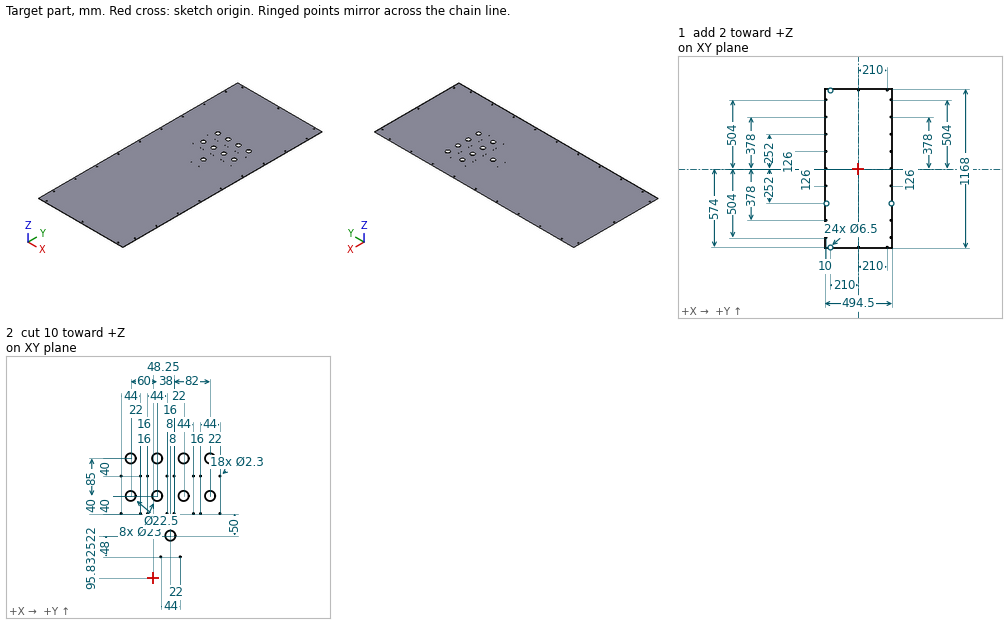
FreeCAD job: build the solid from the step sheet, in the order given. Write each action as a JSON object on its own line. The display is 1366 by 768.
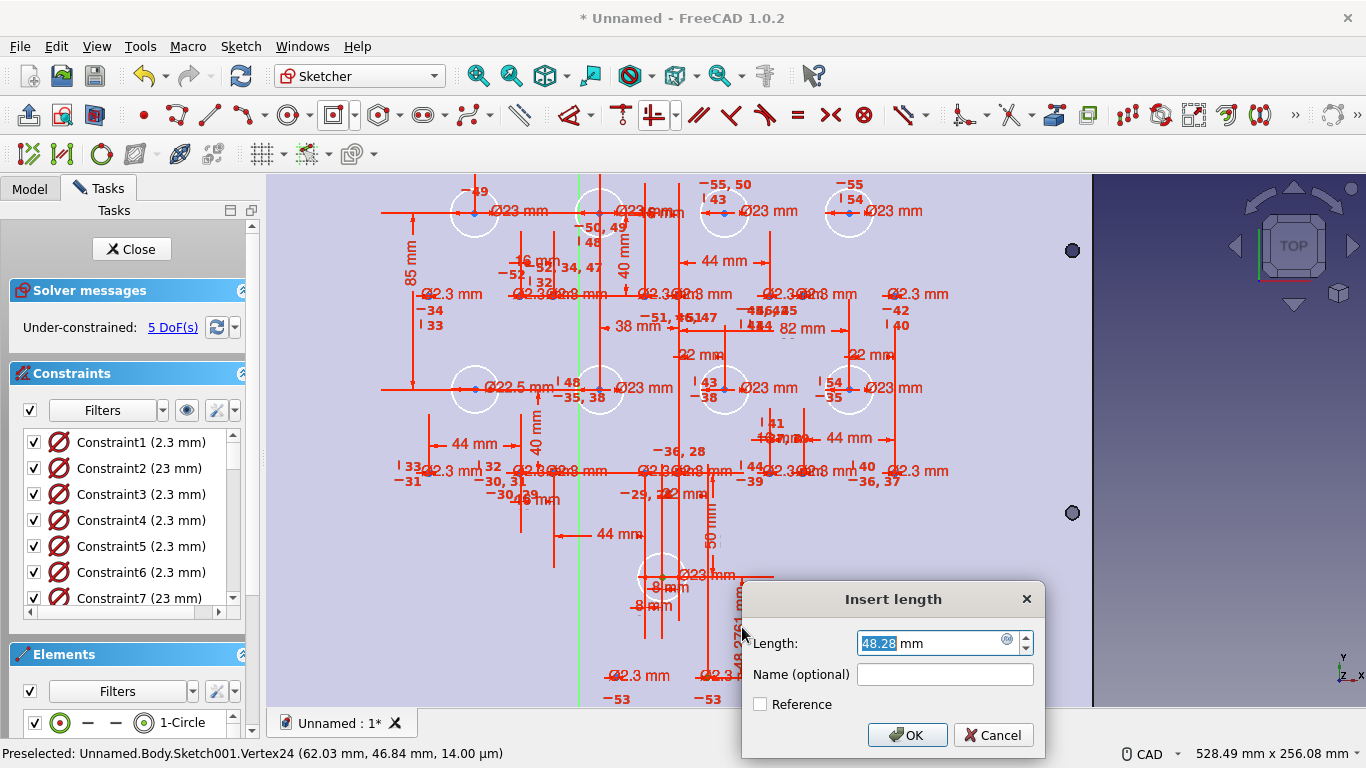
{"action": "type", "text": "48"}
{"action": "key", "text": "Return"}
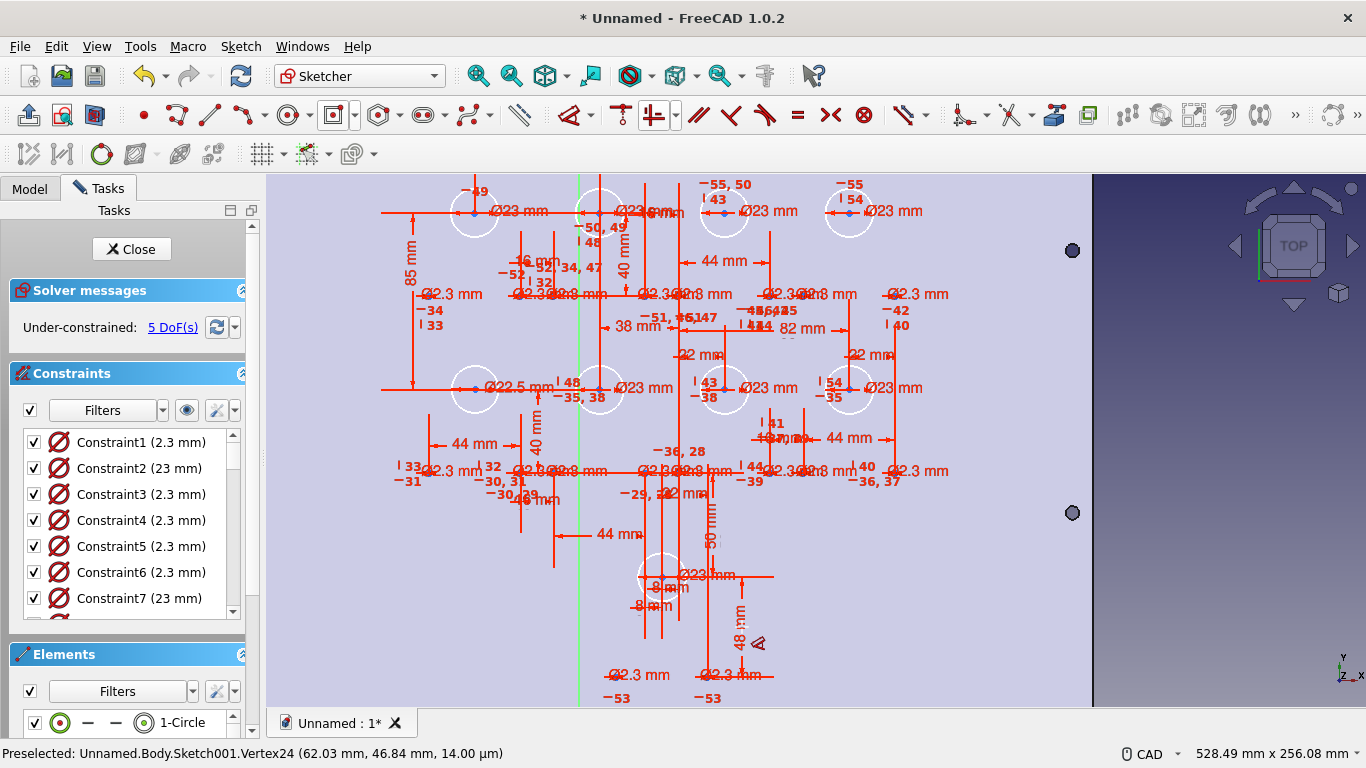
{"action": "left_click", "coordinate": [708, 677]}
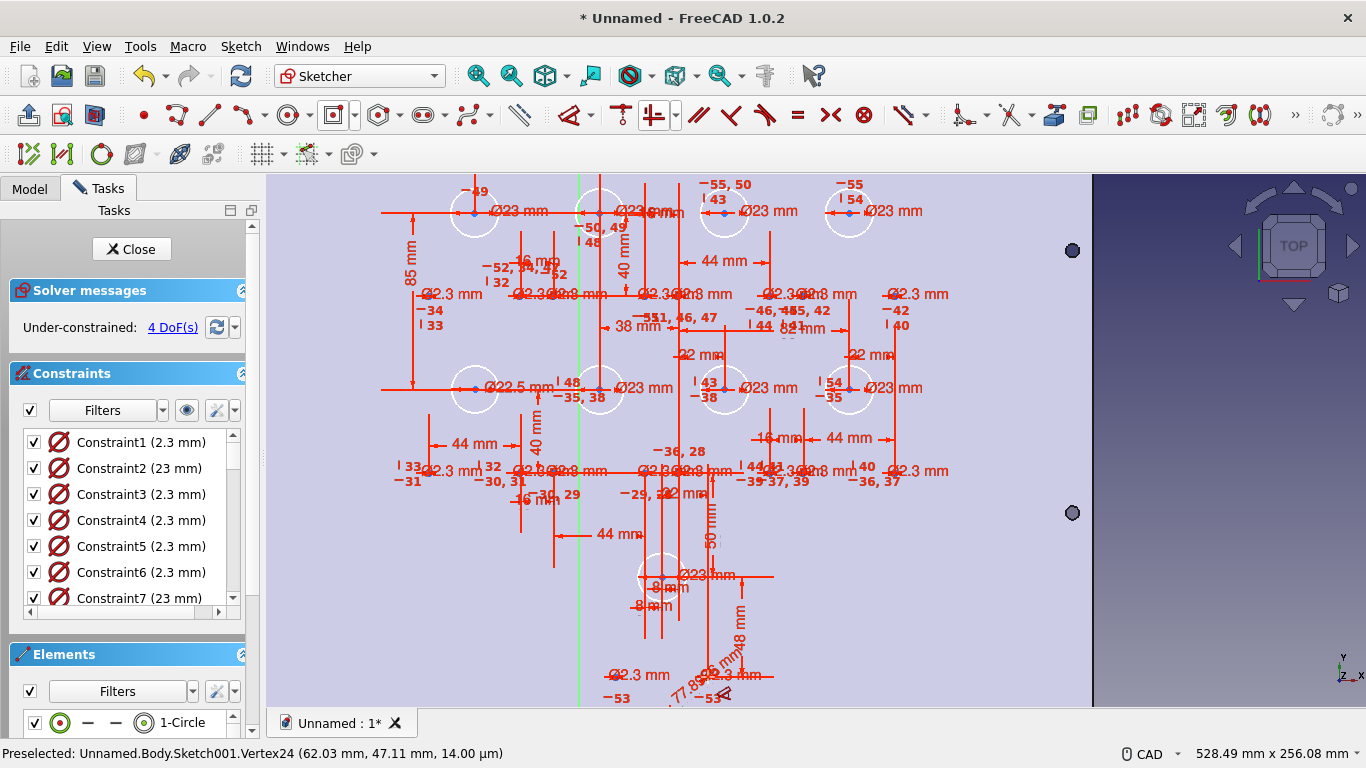
{"action": "left_click", "coordinate": [617, 677]}
{"action": "left_click", "coordinate": [662, 643]}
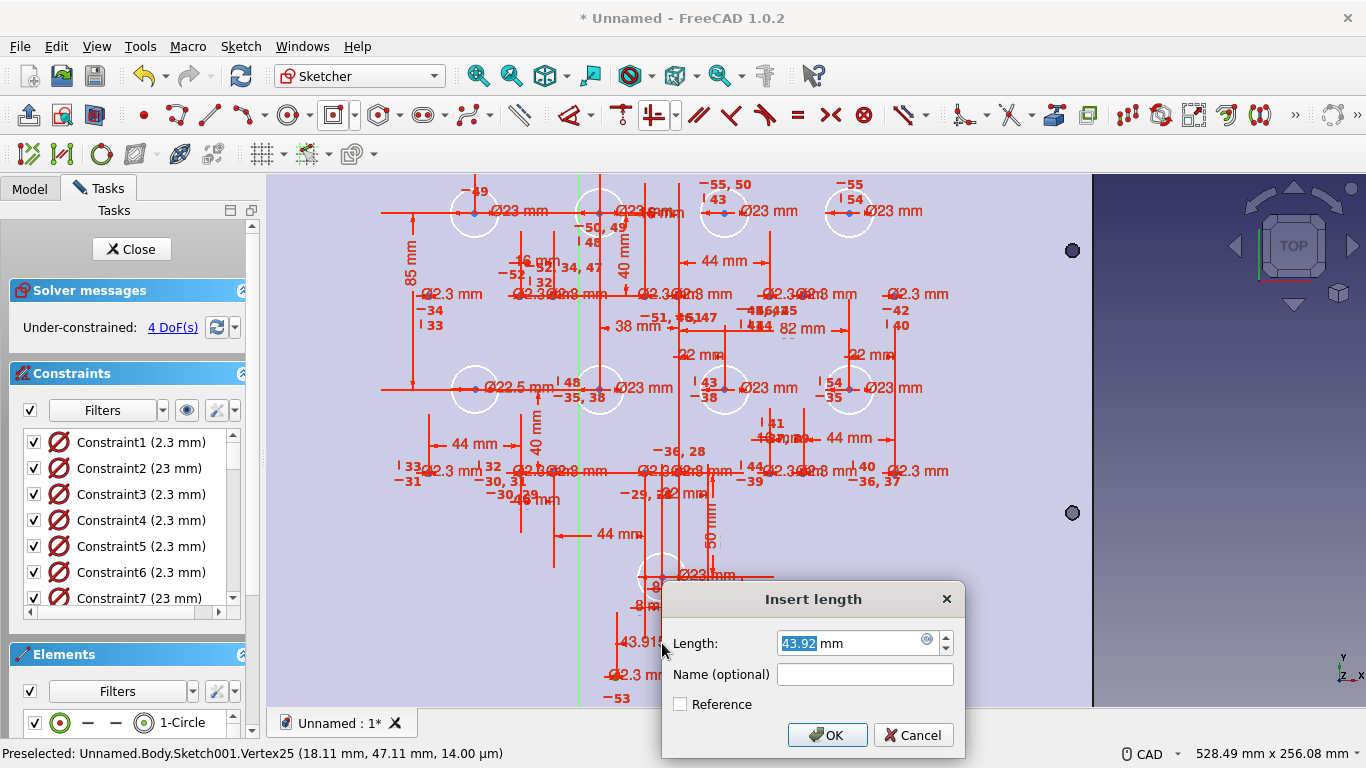
{"action": "type", "text": "44"}
{"action": "key", "text": "Return"}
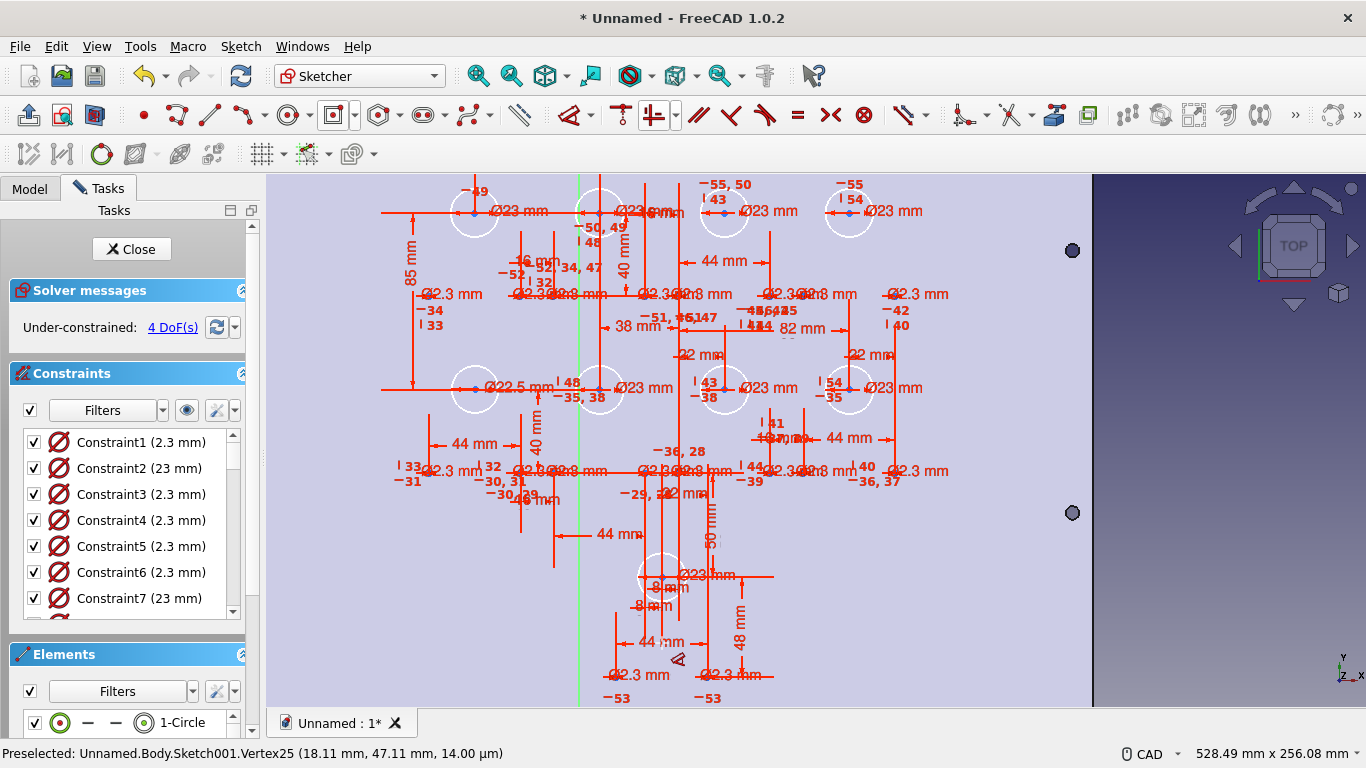
{"action": "left_click", "coordinate": [521, 473]}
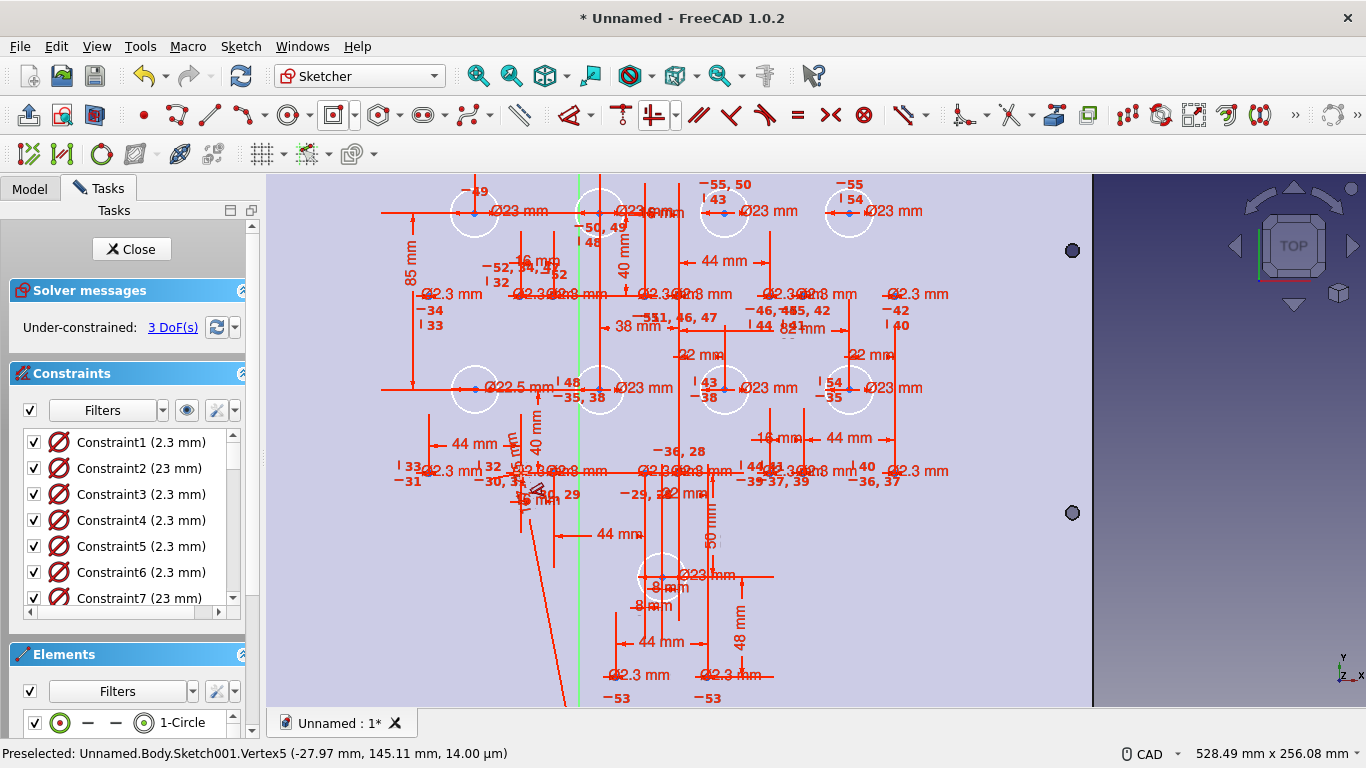
{"action": "left_click", "coordinate": [475, 389]}
{"action": "left_click", "coordinate": [498, 355]}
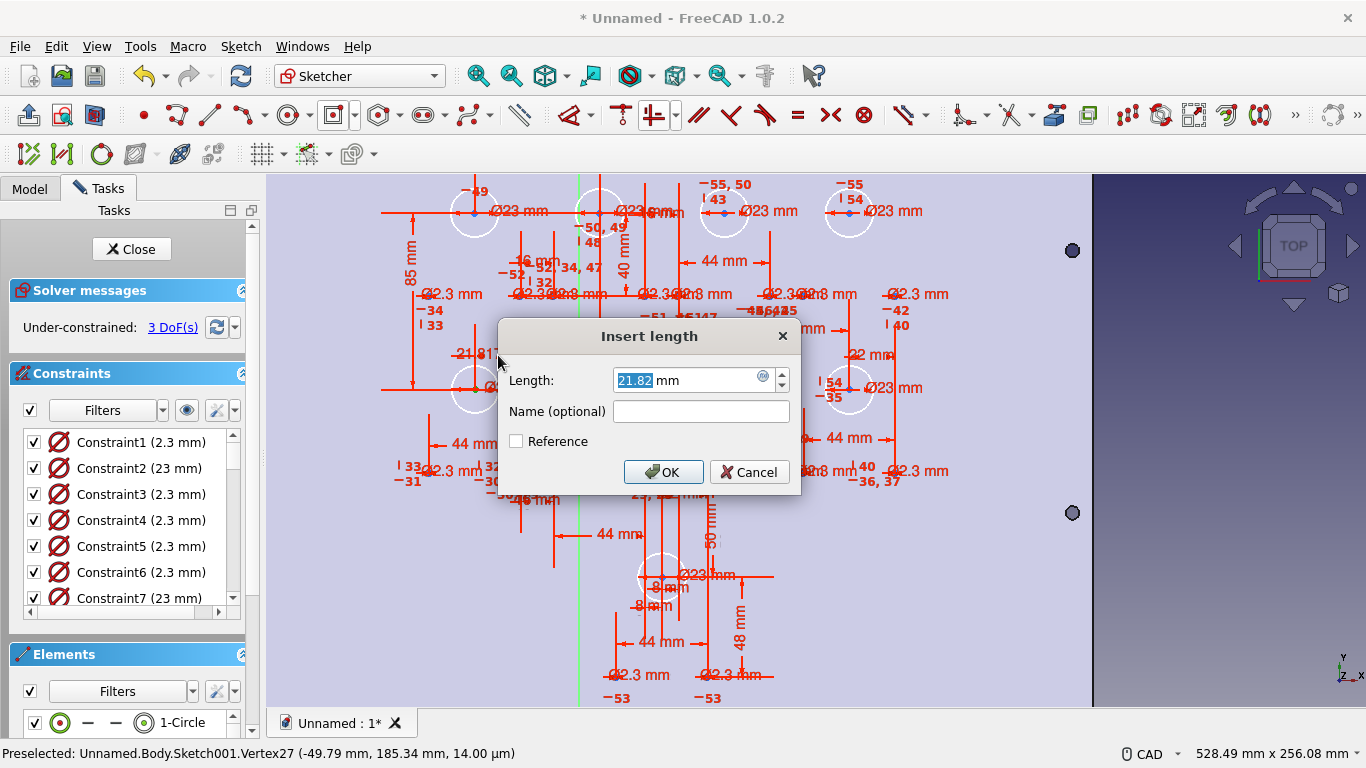
{"action": "type", "text": "22"}
{"action": "key", "text": "Return"}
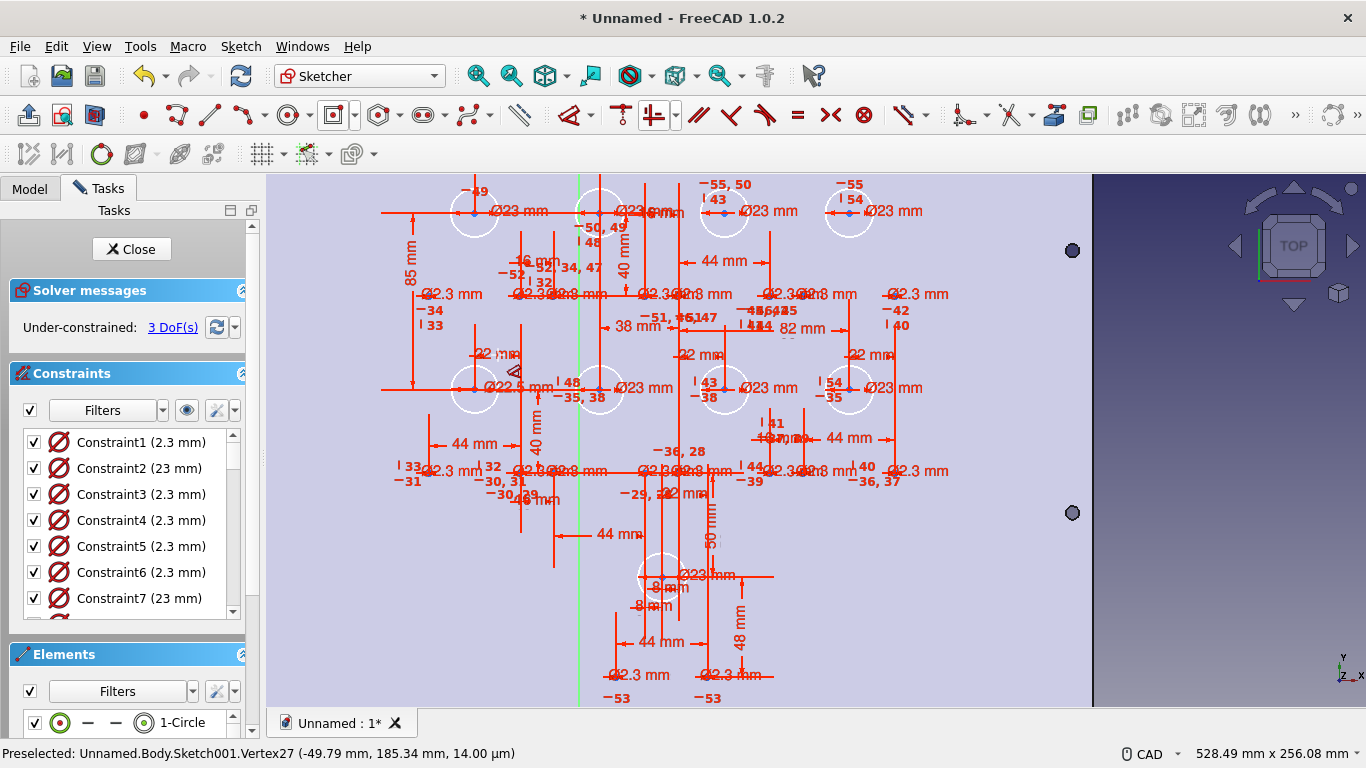
{"action": "left_click", "coordinate": [521, 473]}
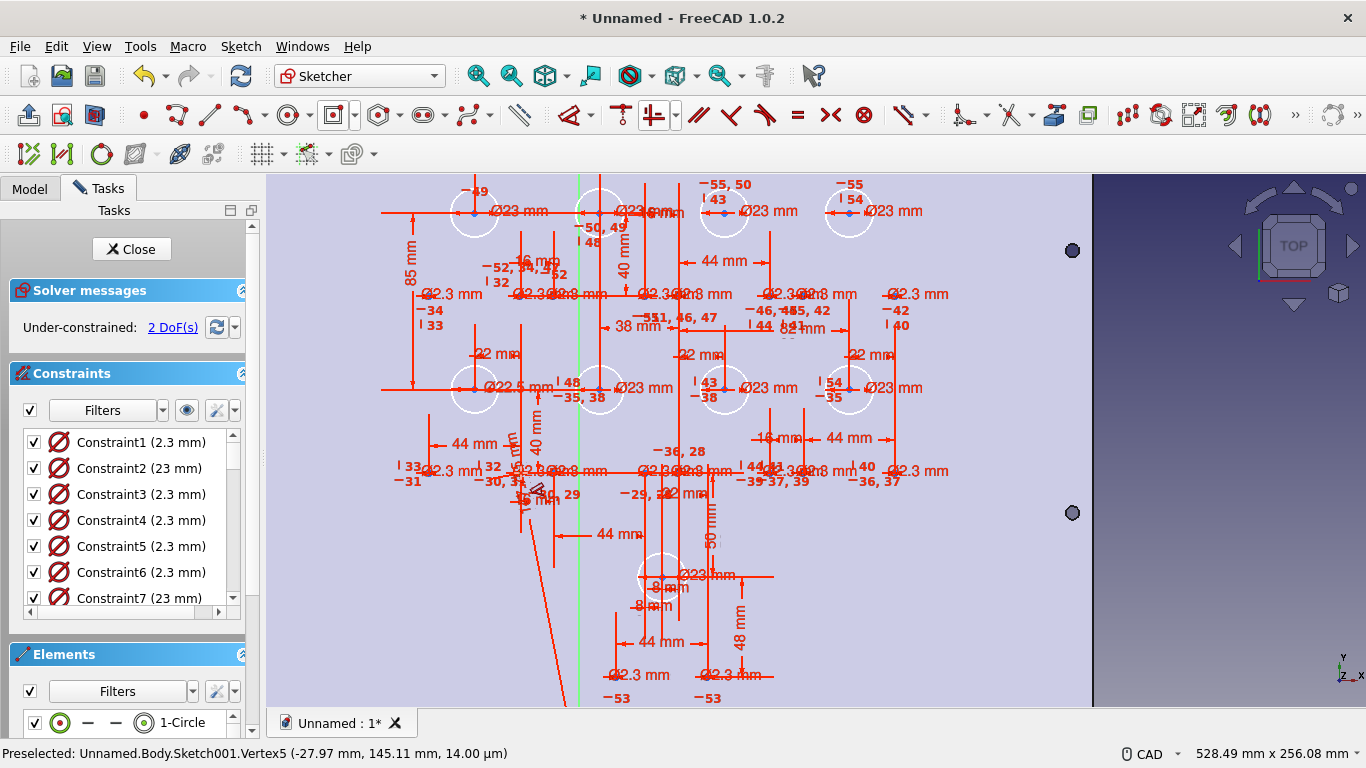
{"action": "left_click", "coordinate": [475, 389]}
{"action": "left_click", "coordinate": [441, 412]}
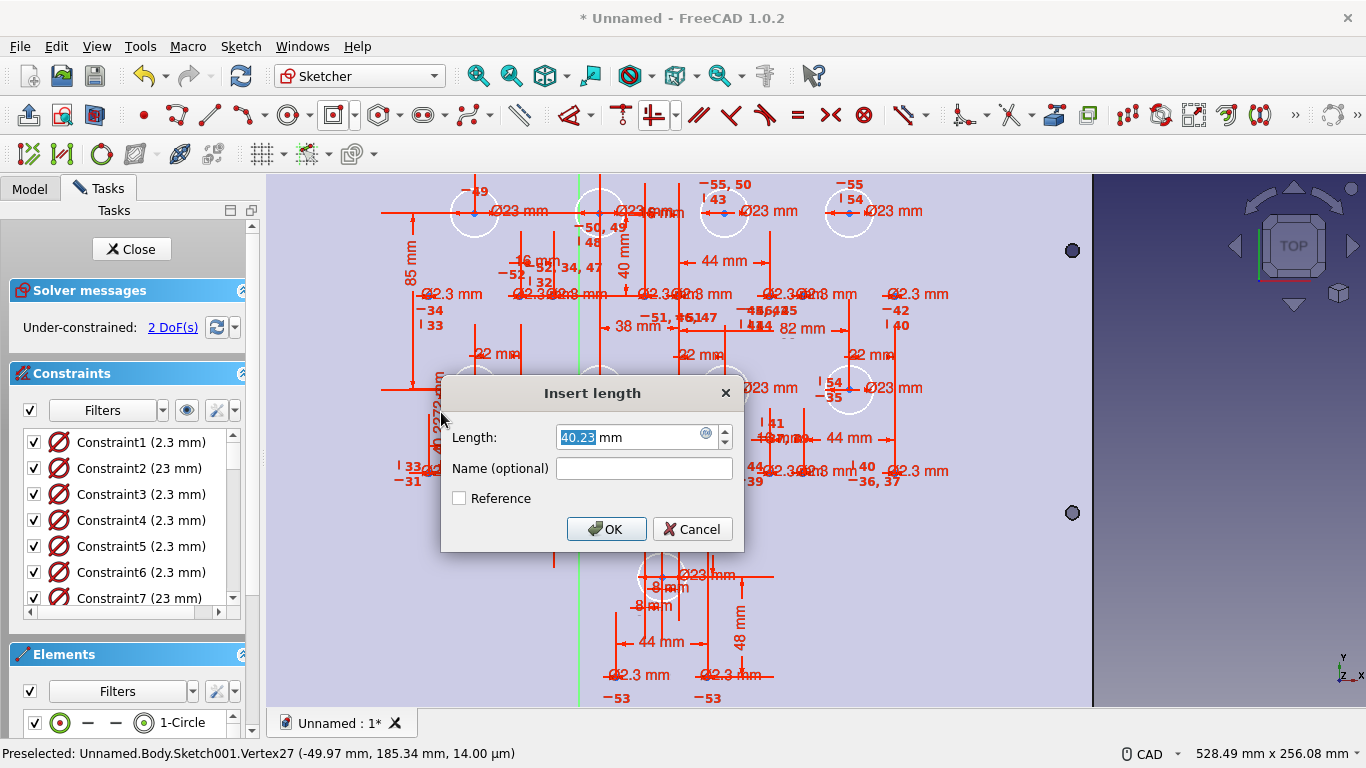
{"action": "type", "text": "40"}
{"action": "key", "text": "Return"}